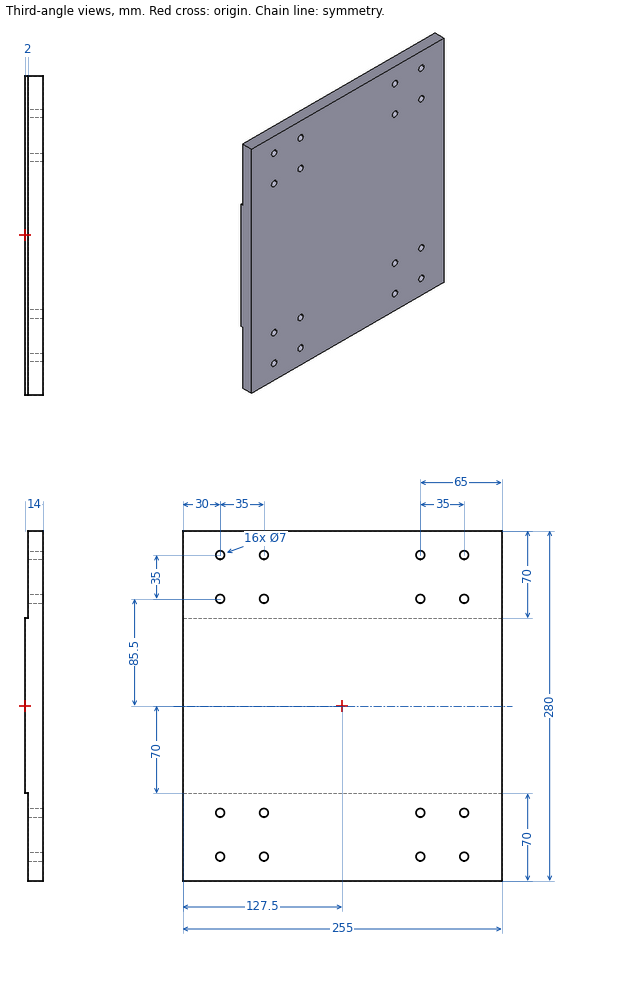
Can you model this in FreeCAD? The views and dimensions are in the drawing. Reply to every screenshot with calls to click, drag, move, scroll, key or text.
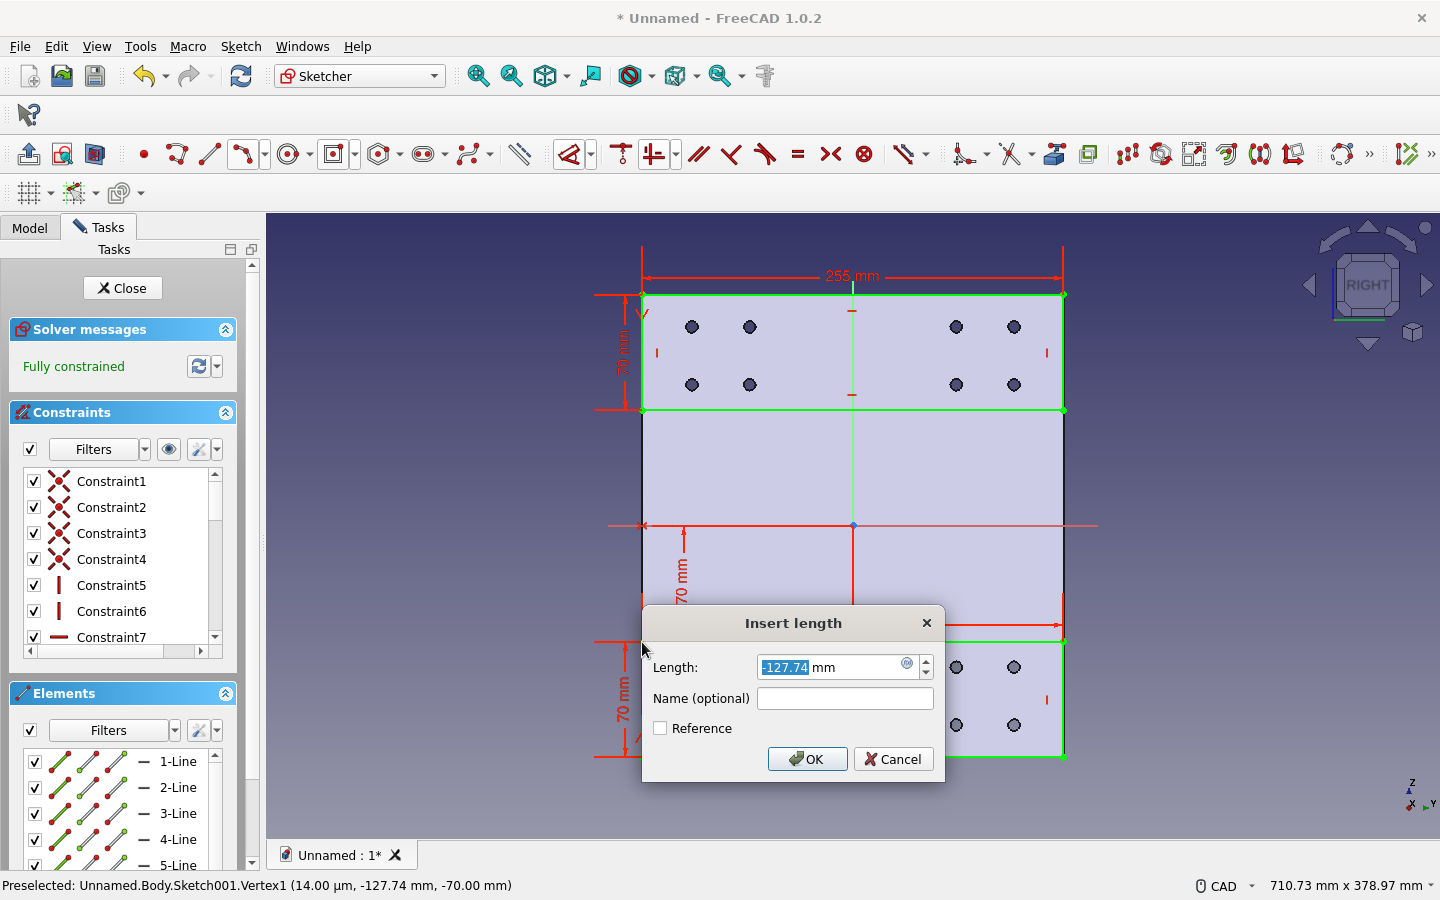
text(-127.5)
key(Return)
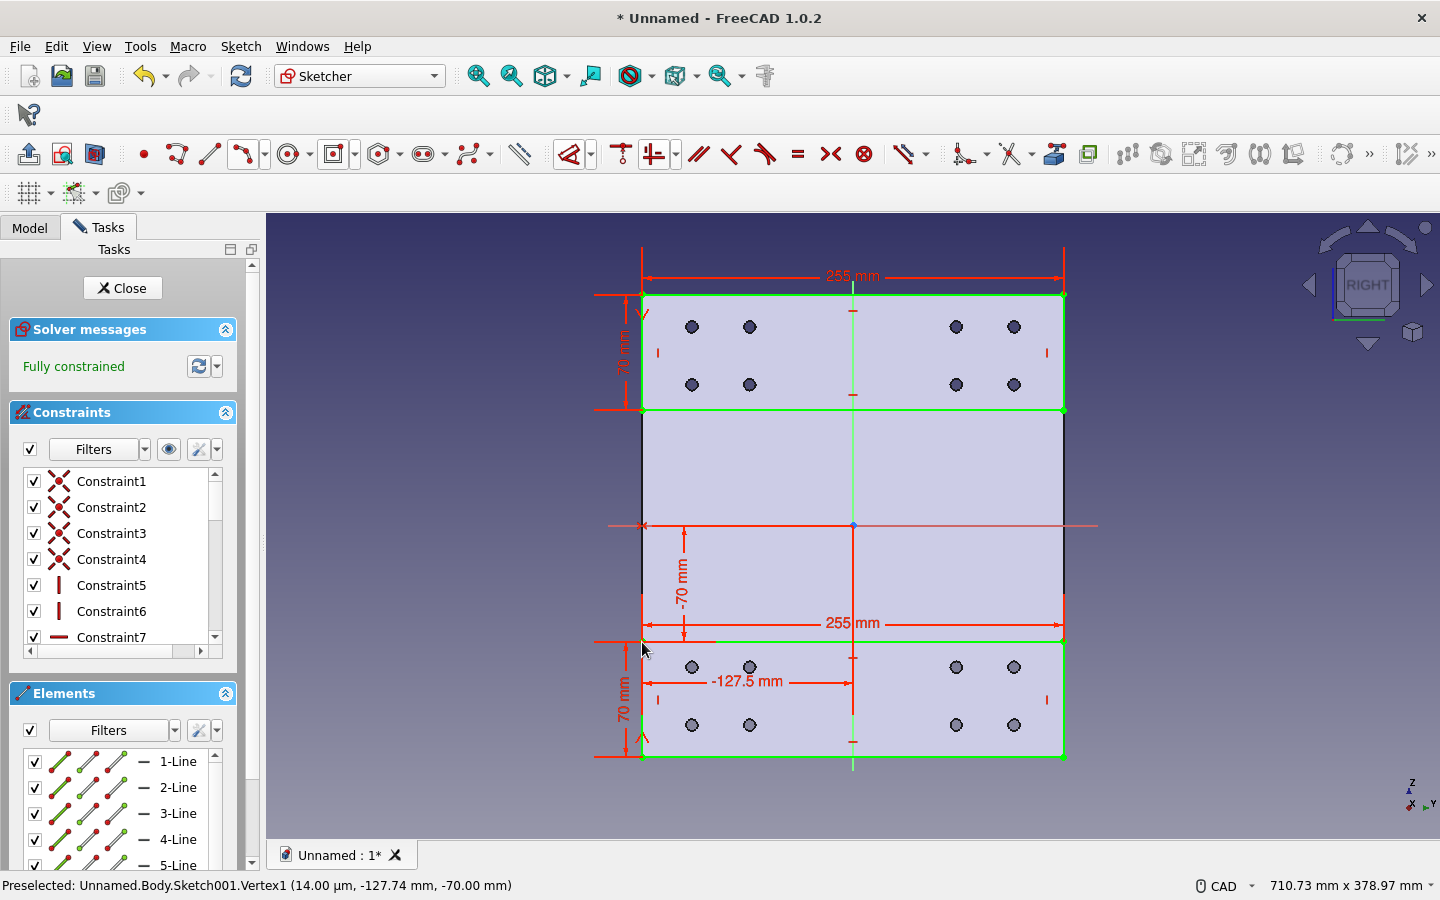
click(123, 288)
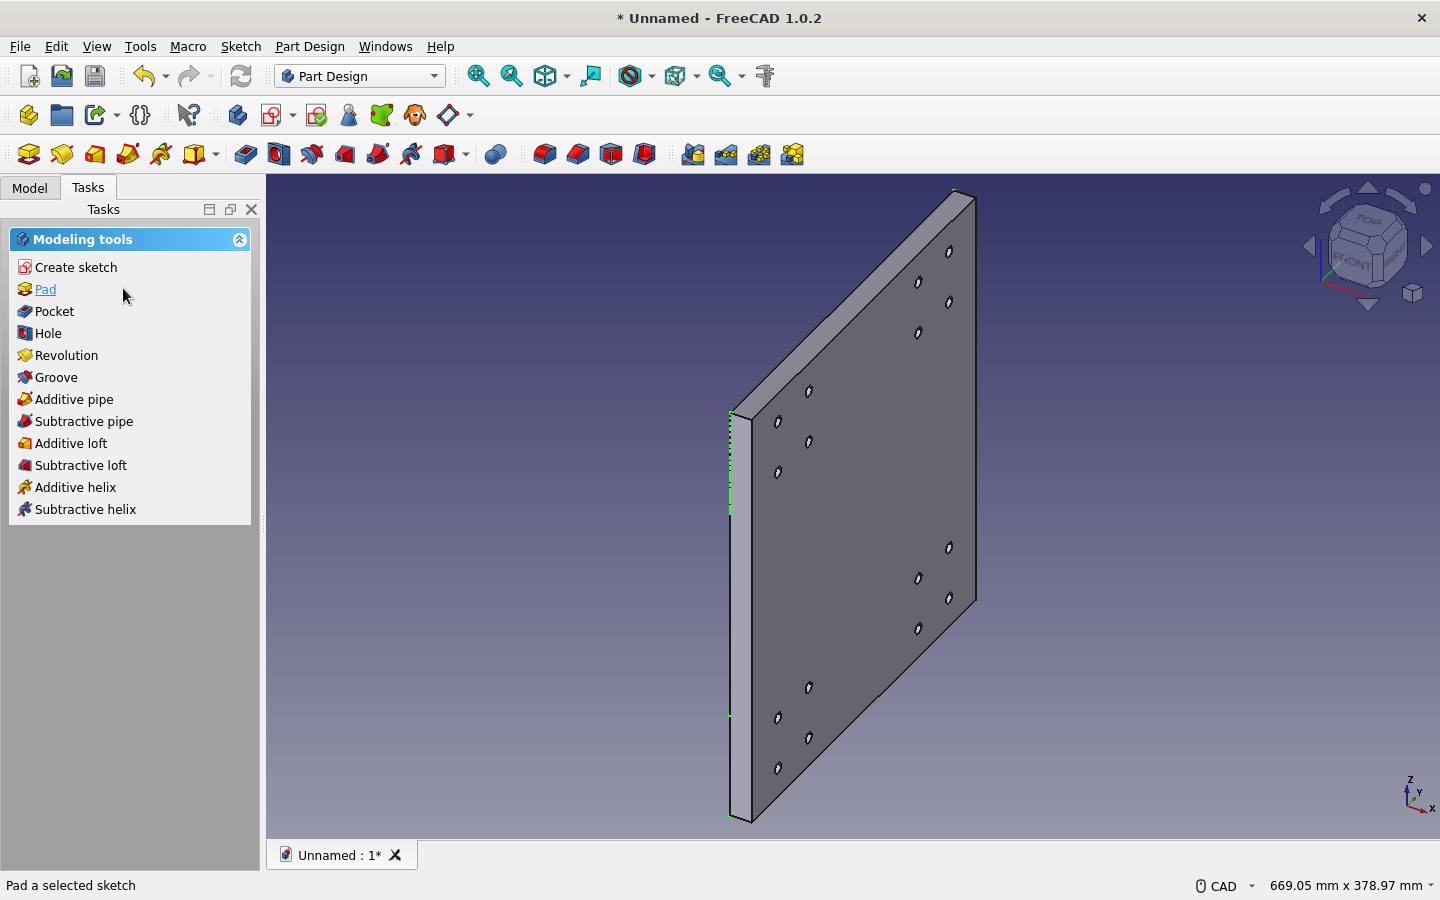
click(246, 154)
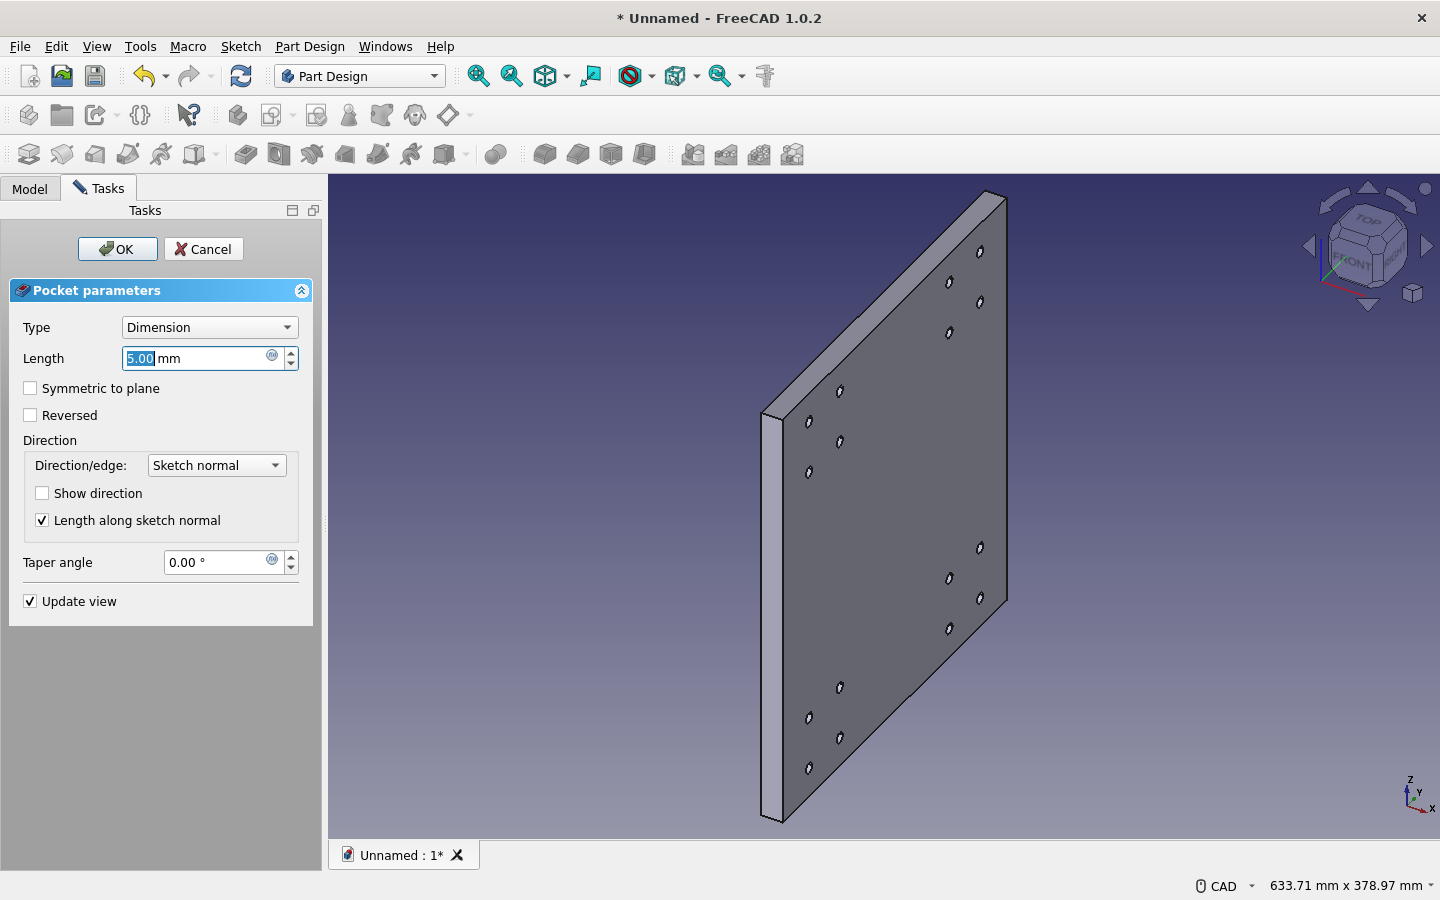
text(2)
key(Tab)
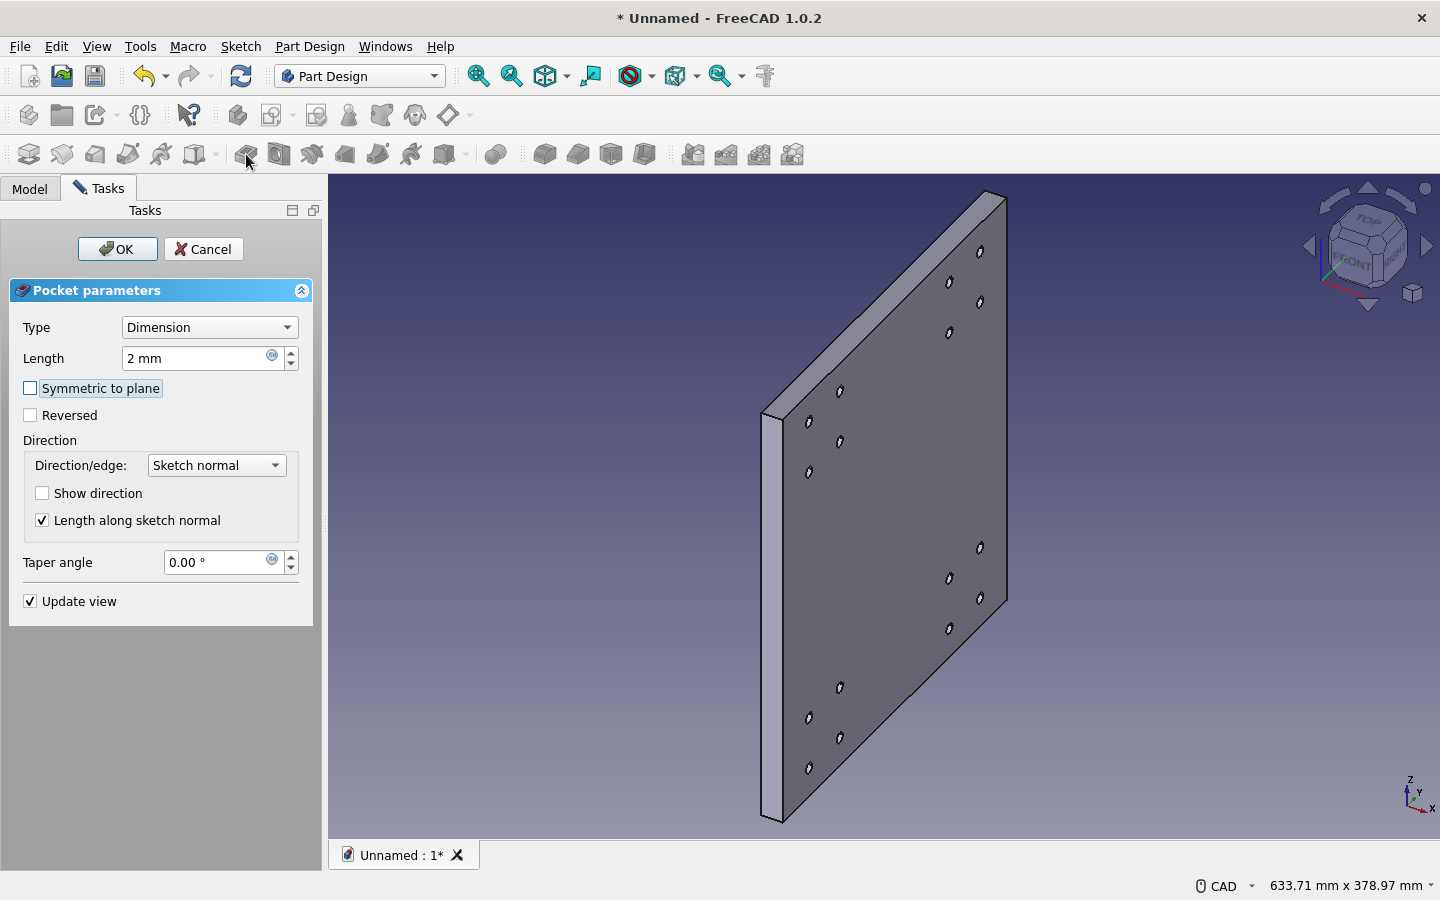
click(31, 415)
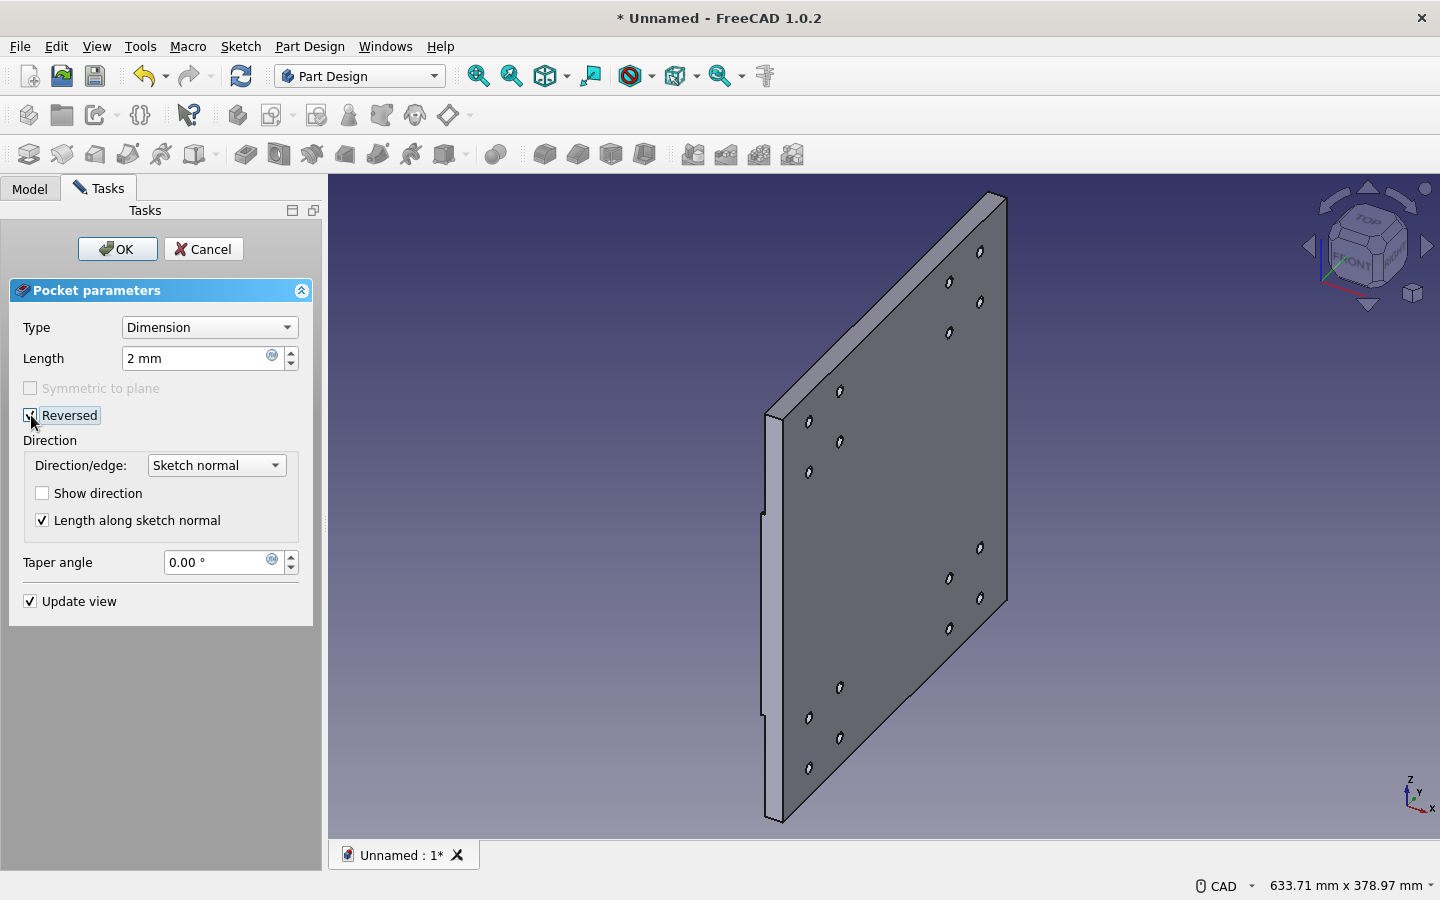
click(118, 249)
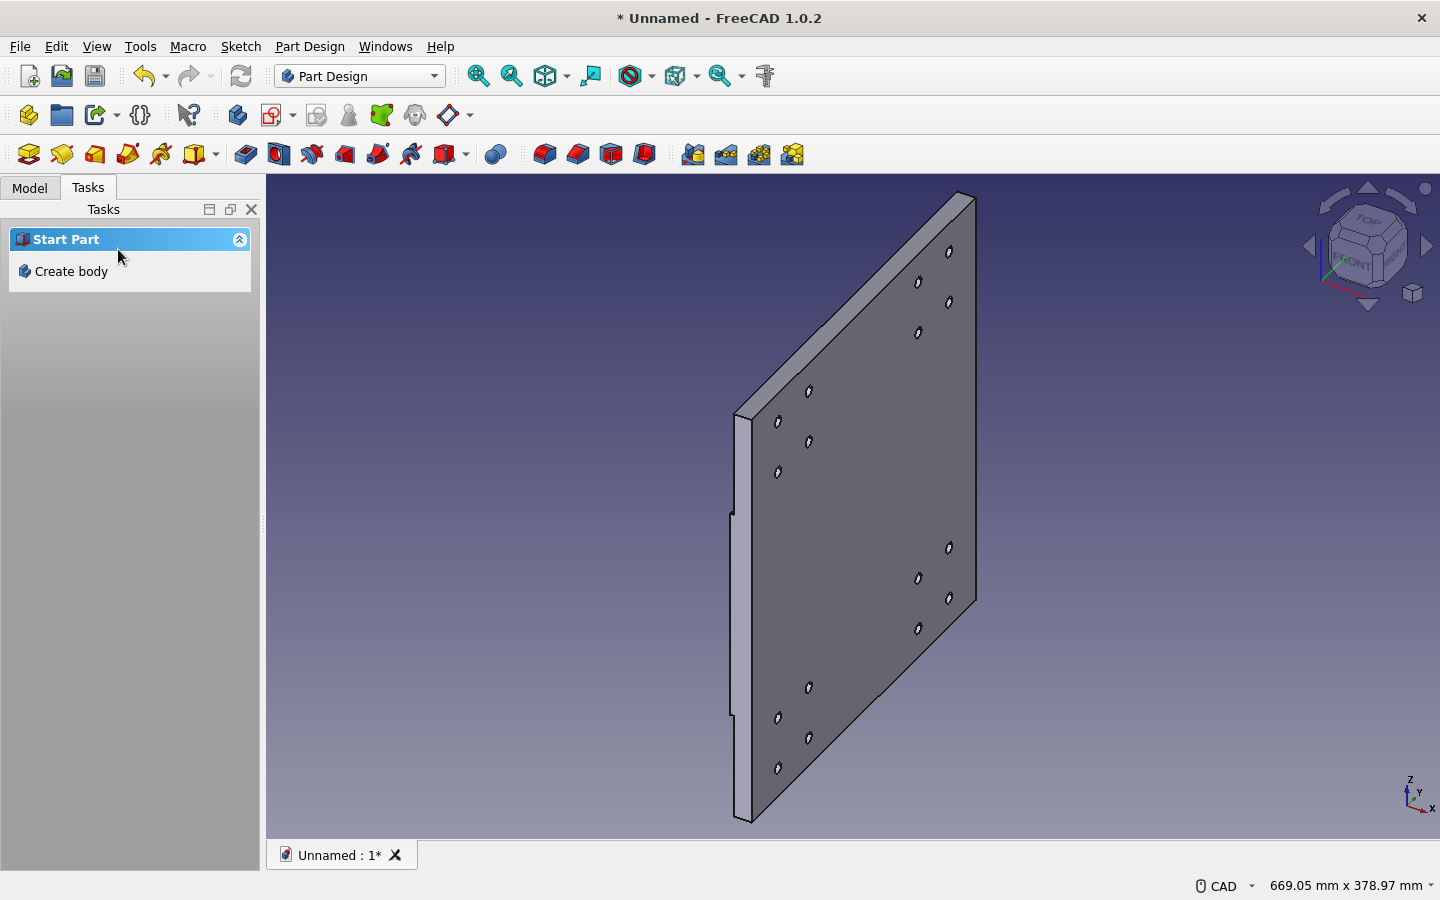
key(0)